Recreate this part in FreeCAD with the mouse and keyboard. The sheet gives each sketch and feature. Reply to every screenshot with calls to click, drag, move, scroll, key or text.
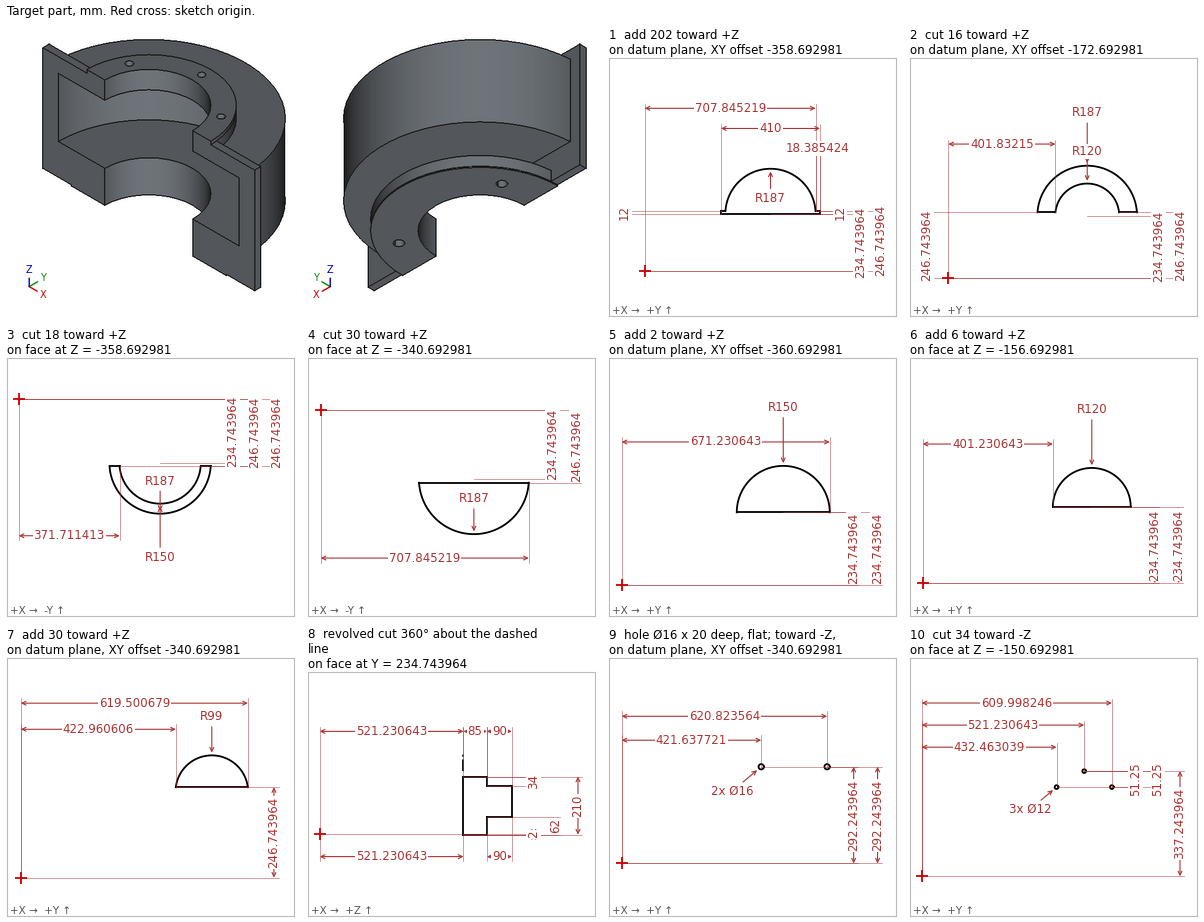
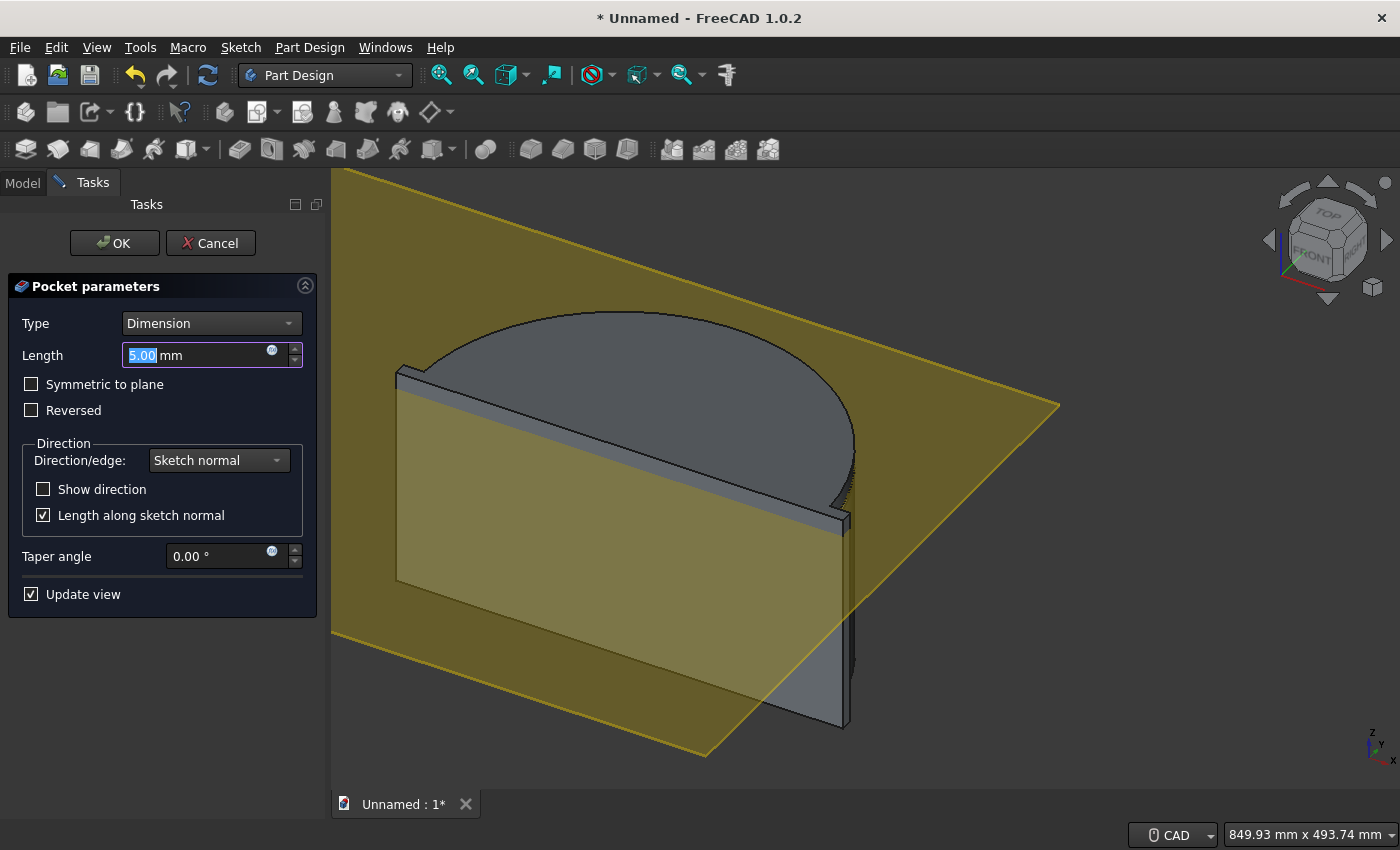
text(16)
key(Tab)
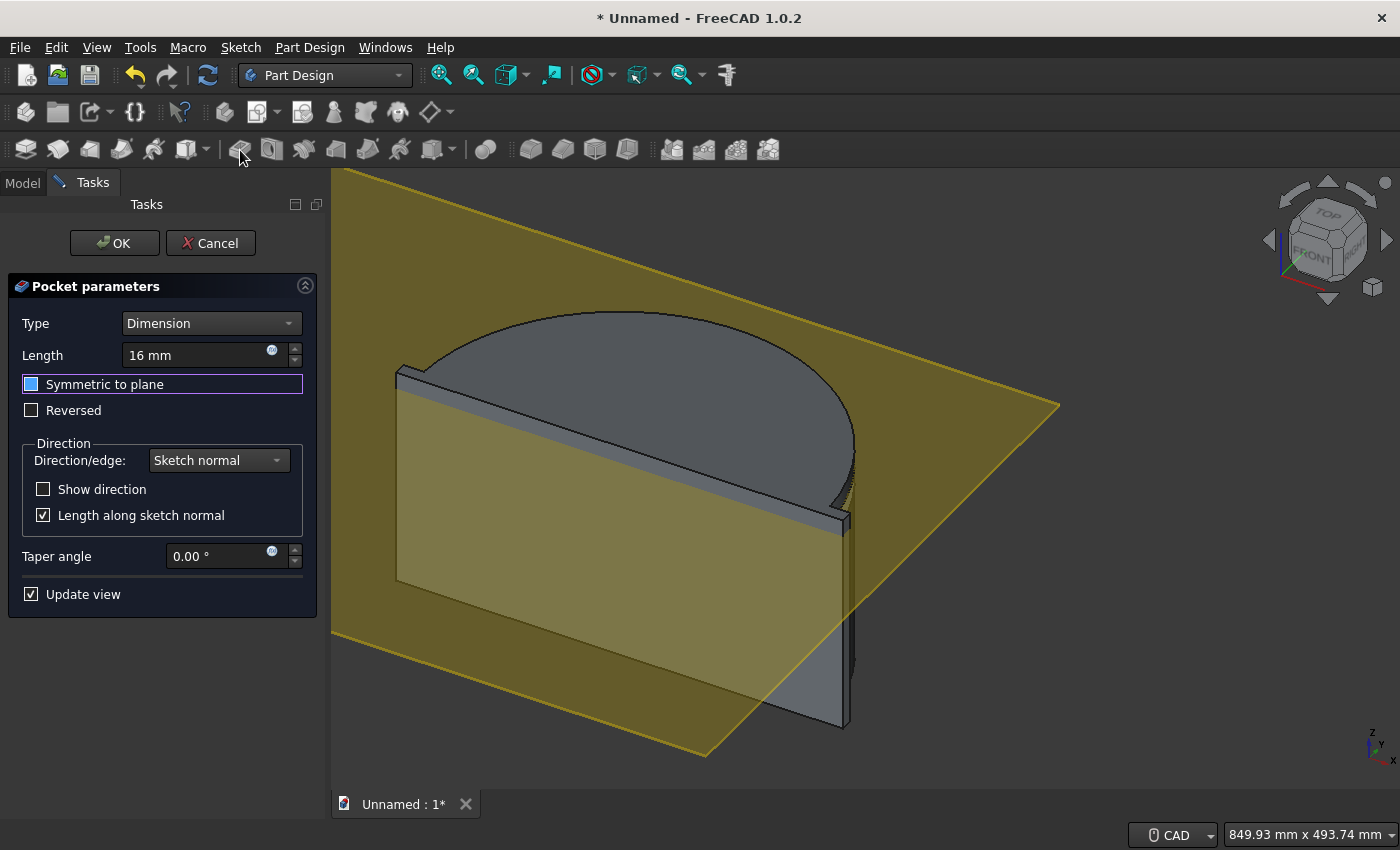
click(30, 410)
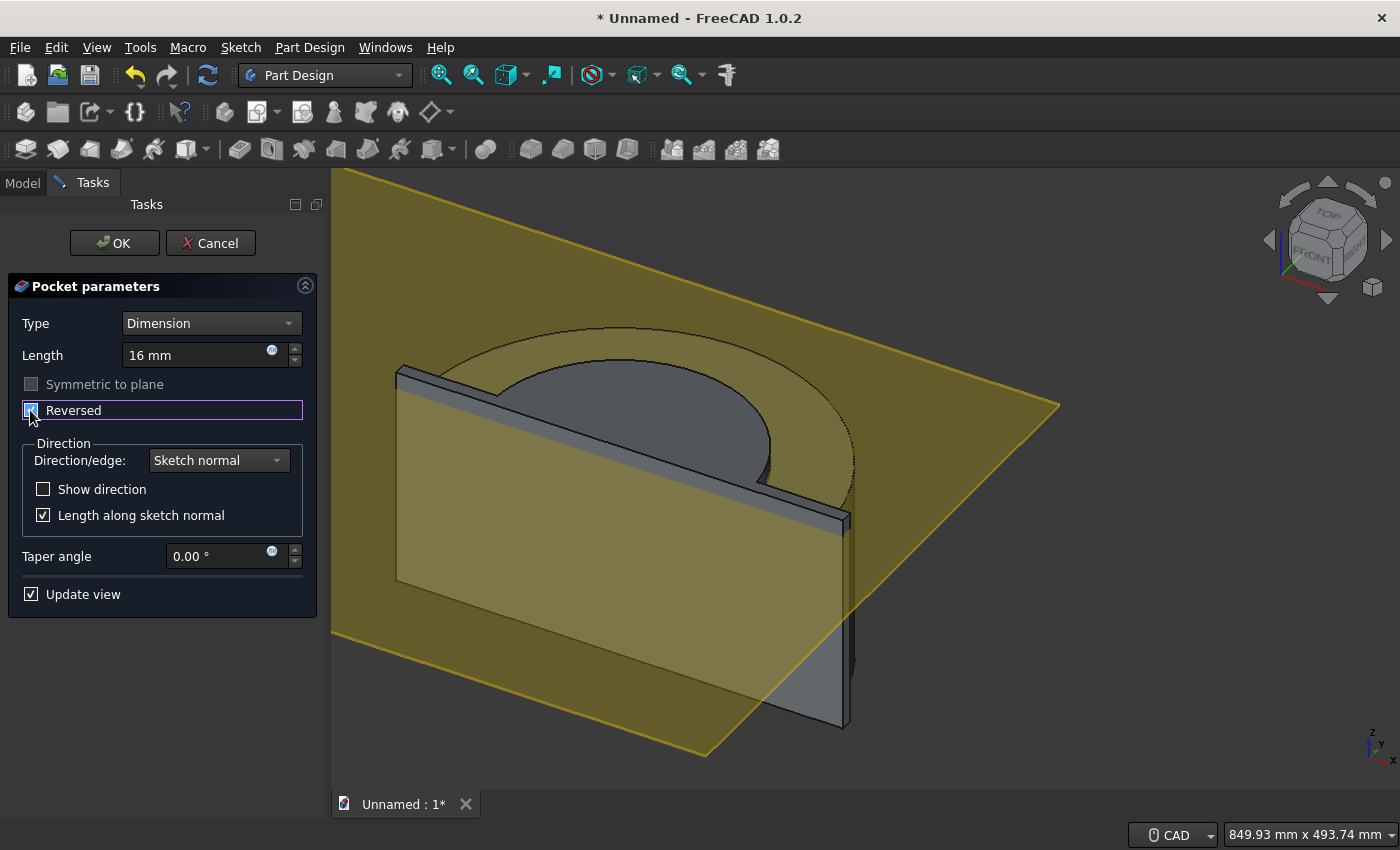
click(115, 243)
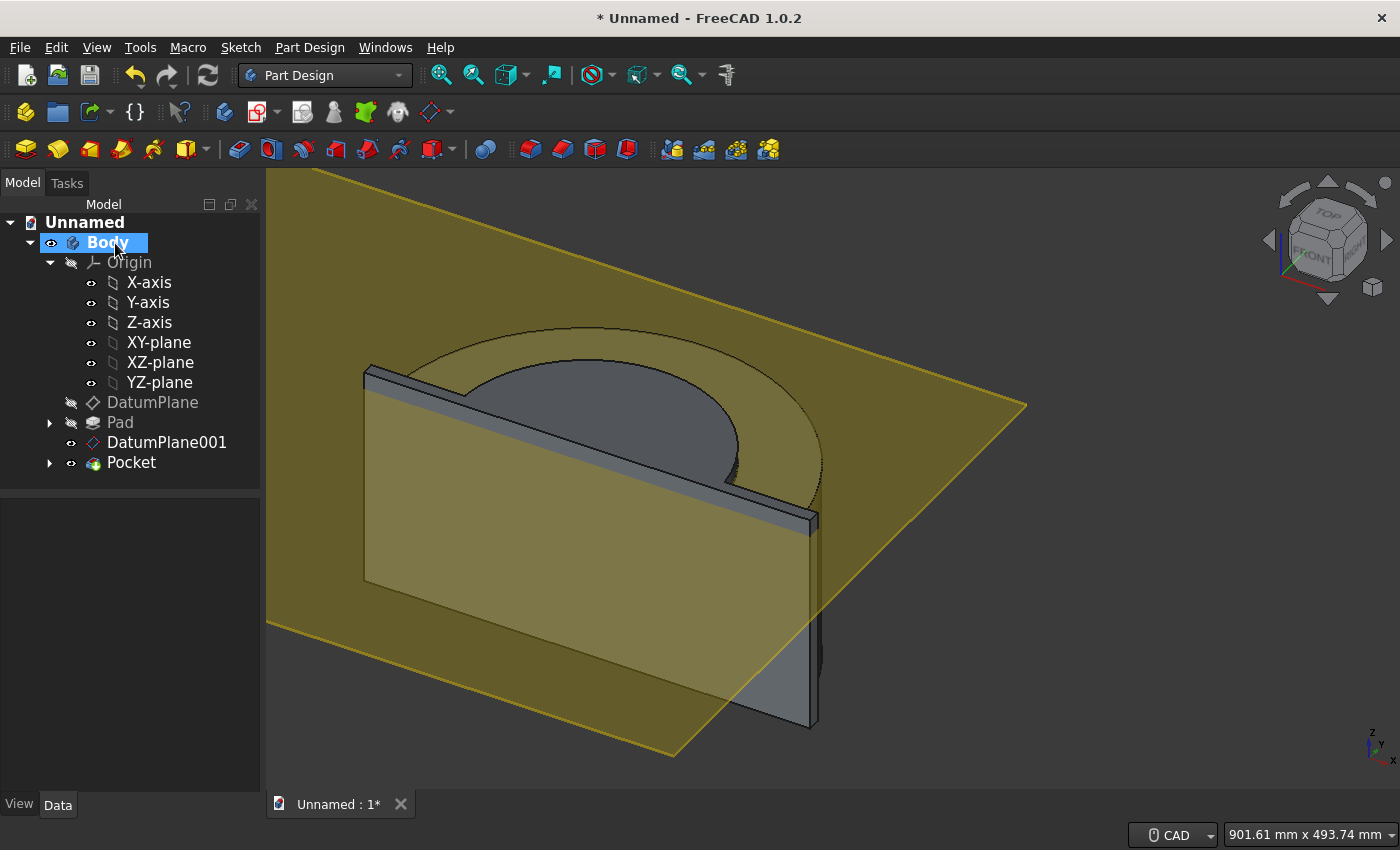
click(116, 443)
key(space)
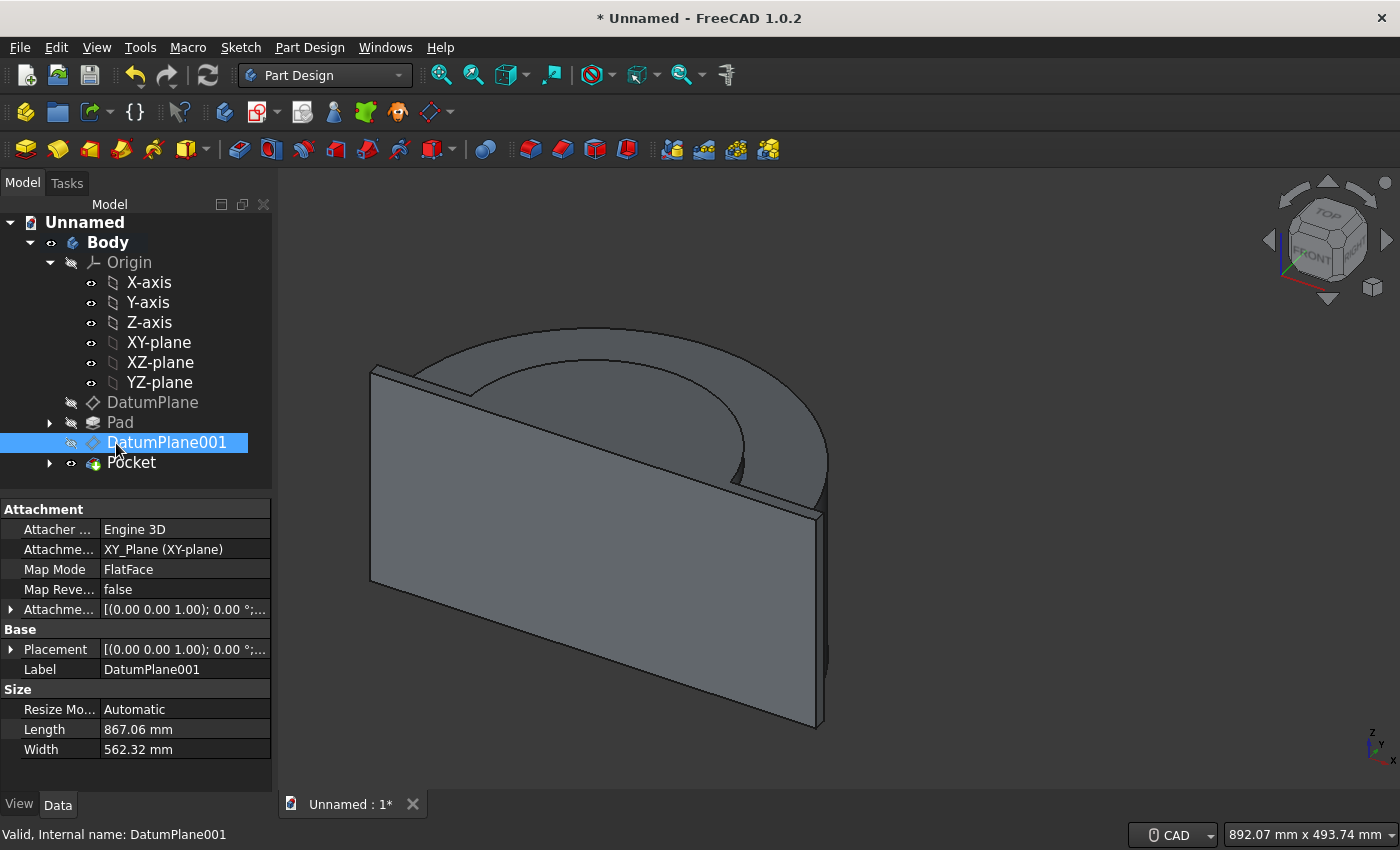
key(5)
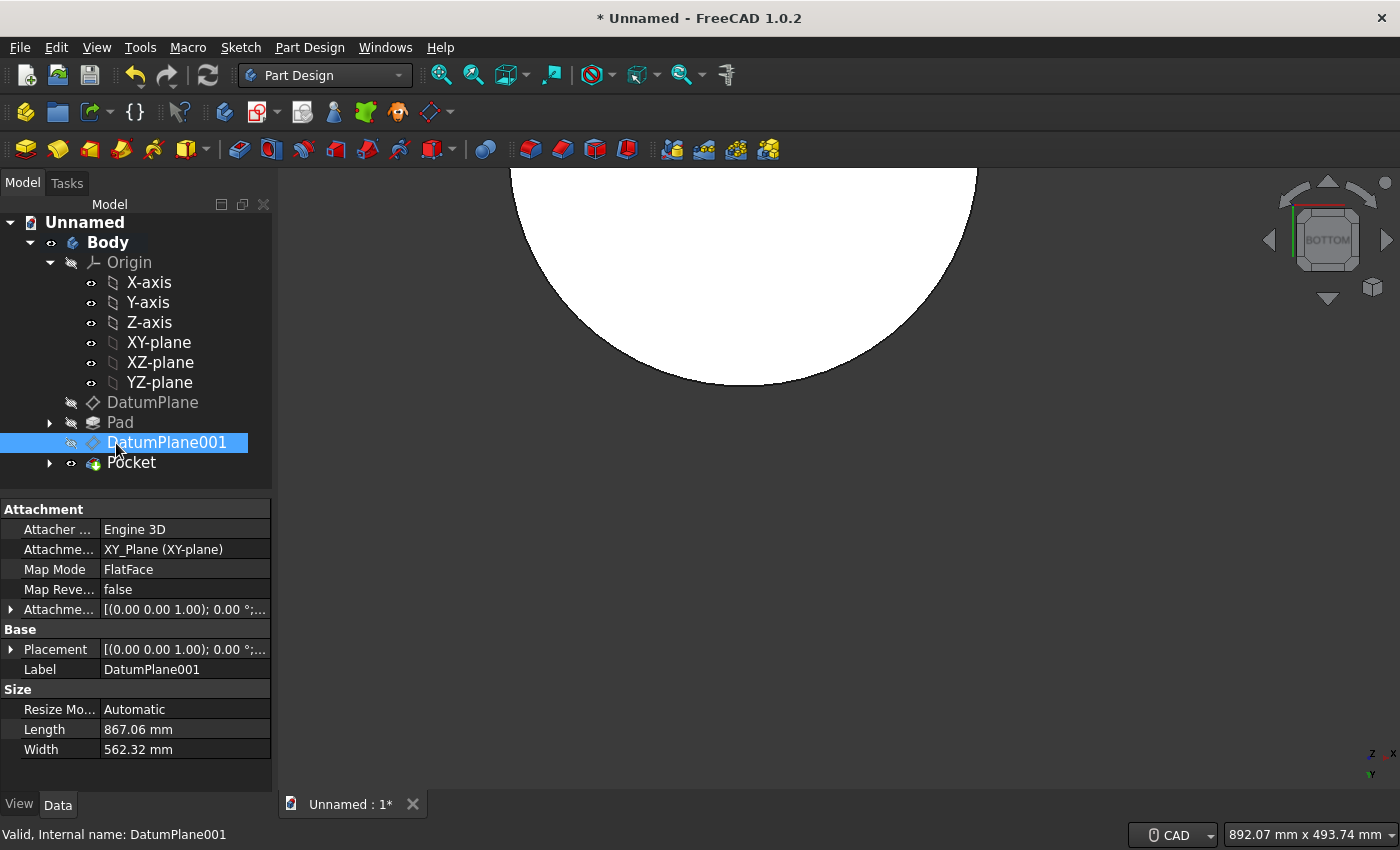
click(442, 76)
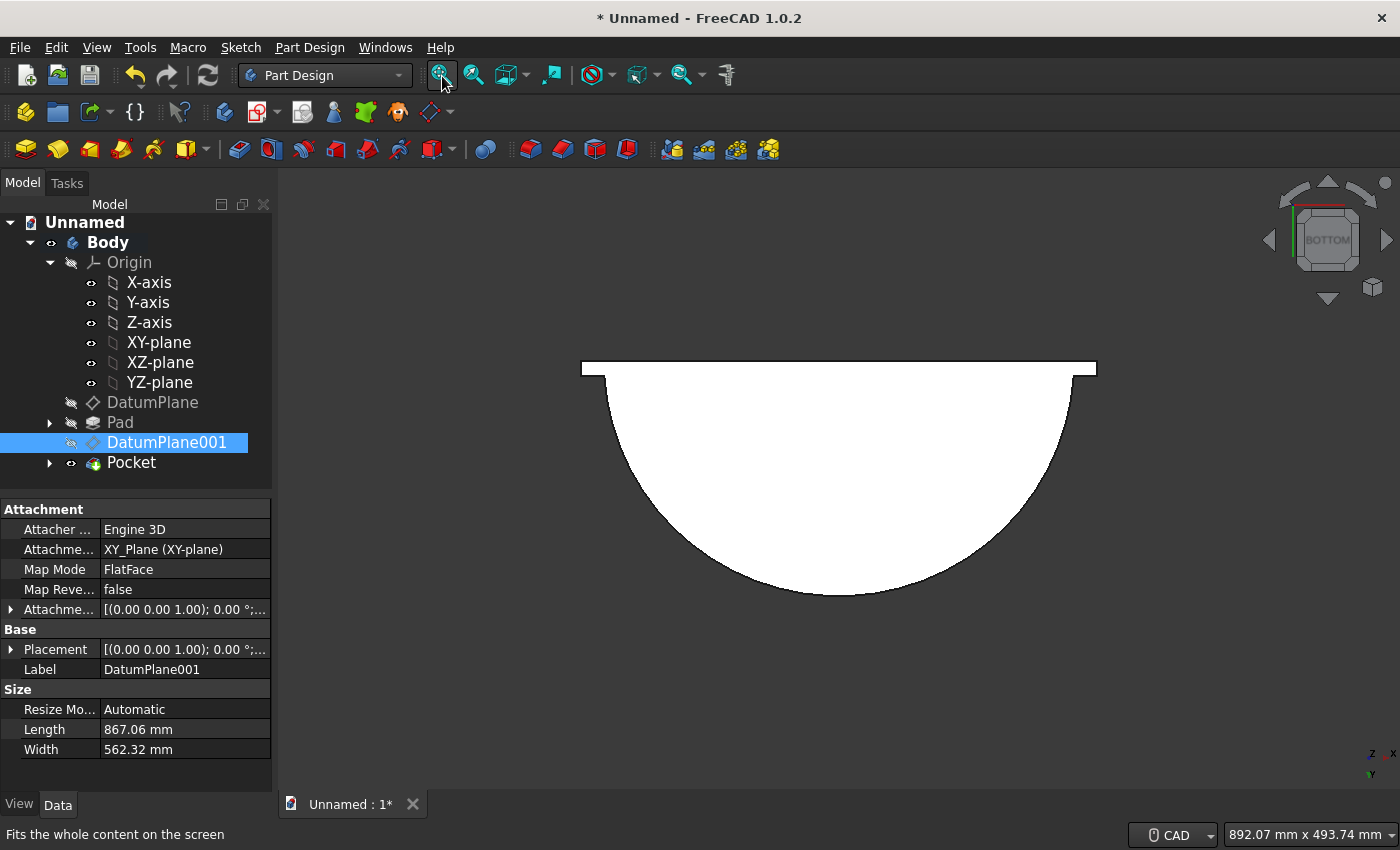
click(839, 478)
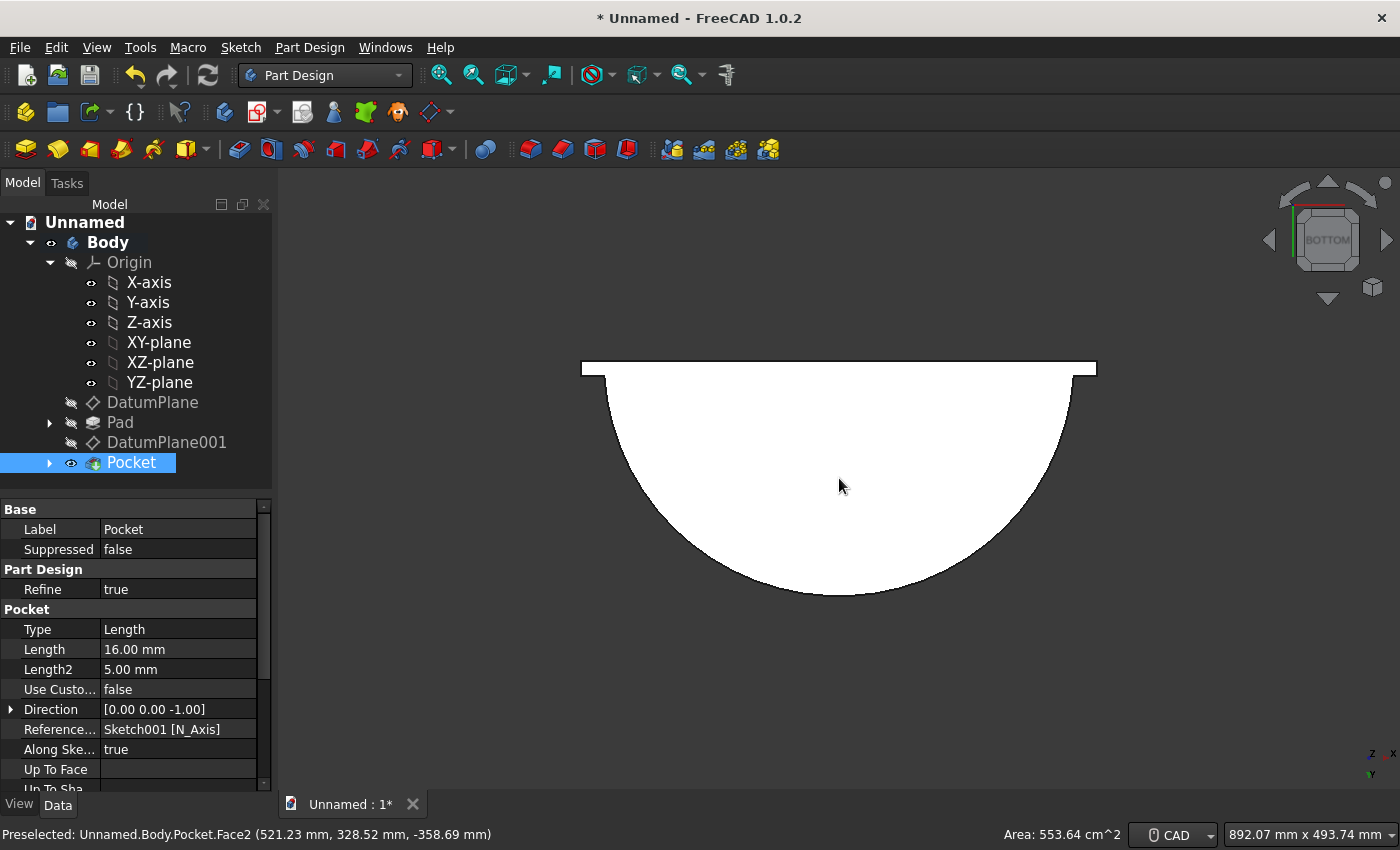
click(258, 112)